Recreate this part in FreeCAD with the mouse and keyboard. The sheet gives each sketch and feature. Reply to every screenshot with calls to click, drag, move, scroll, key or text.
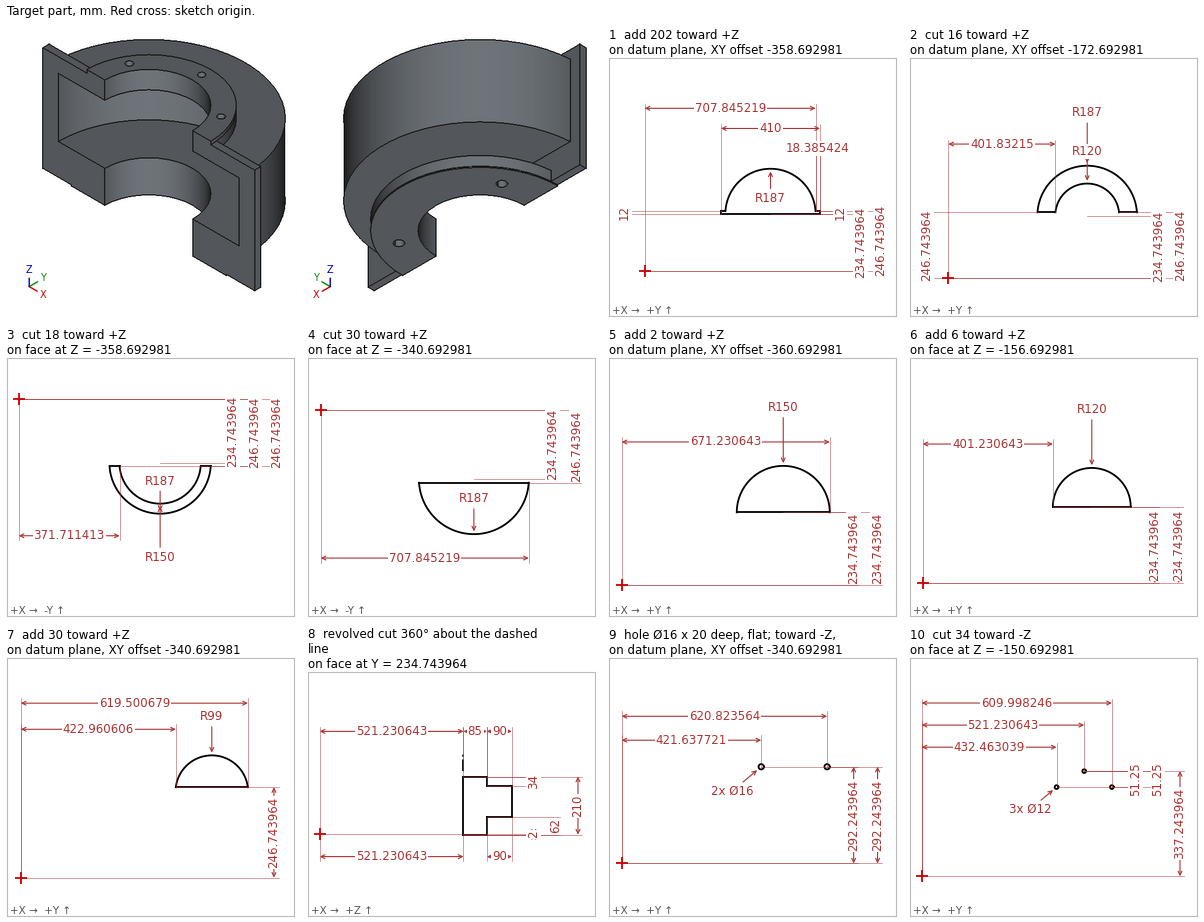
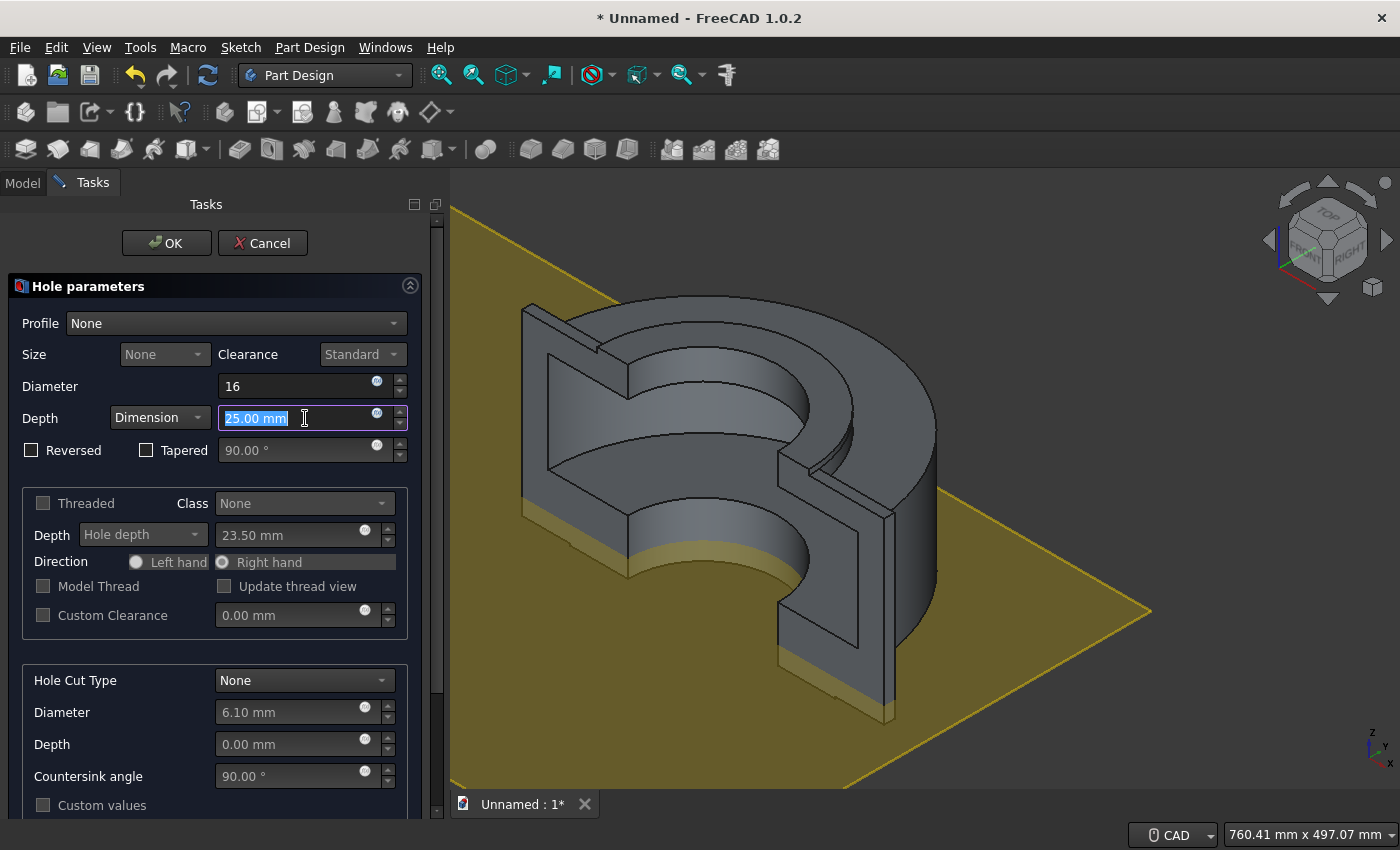
text(20)
key(Tab)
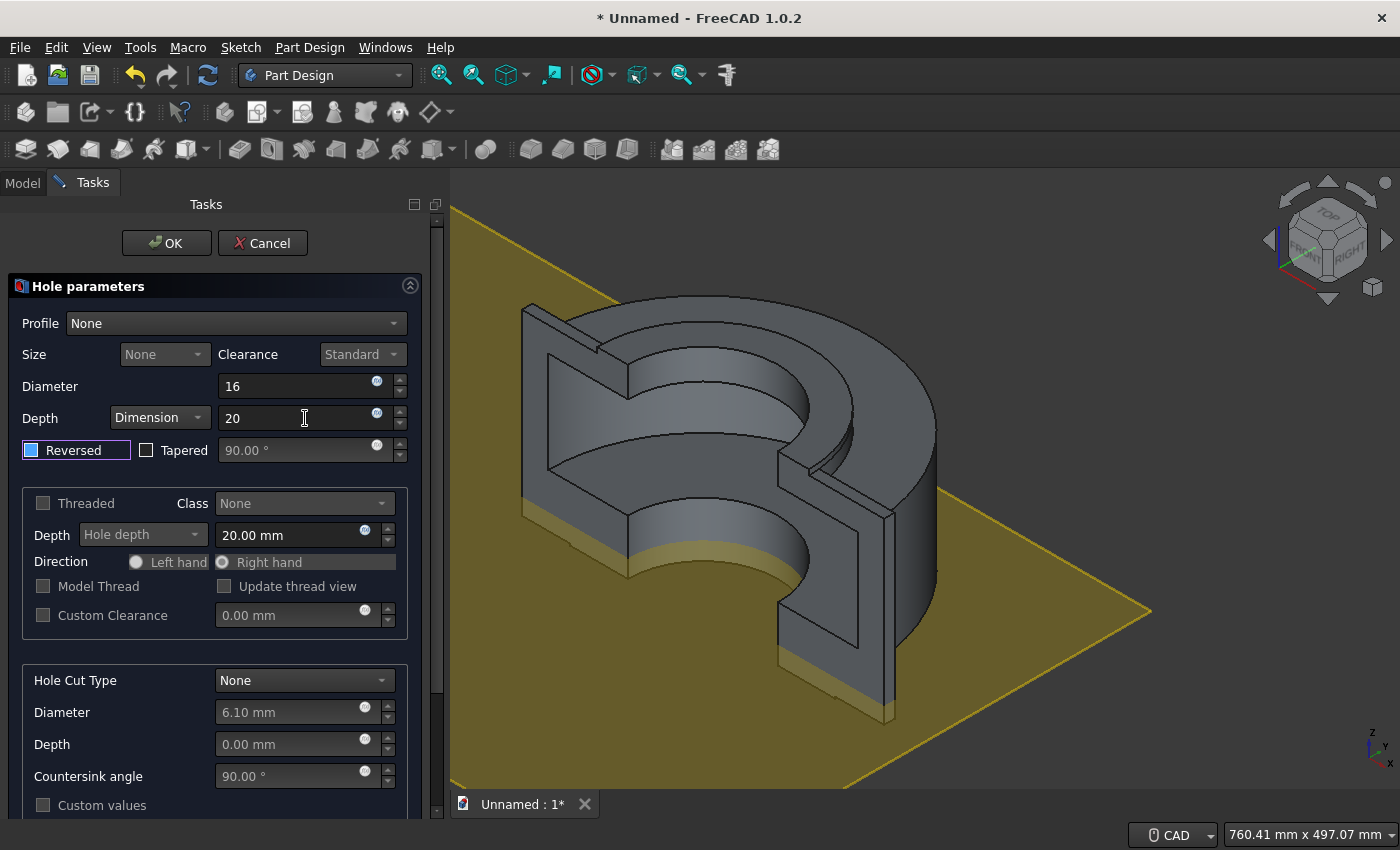
scroll(437, 516, down, 2)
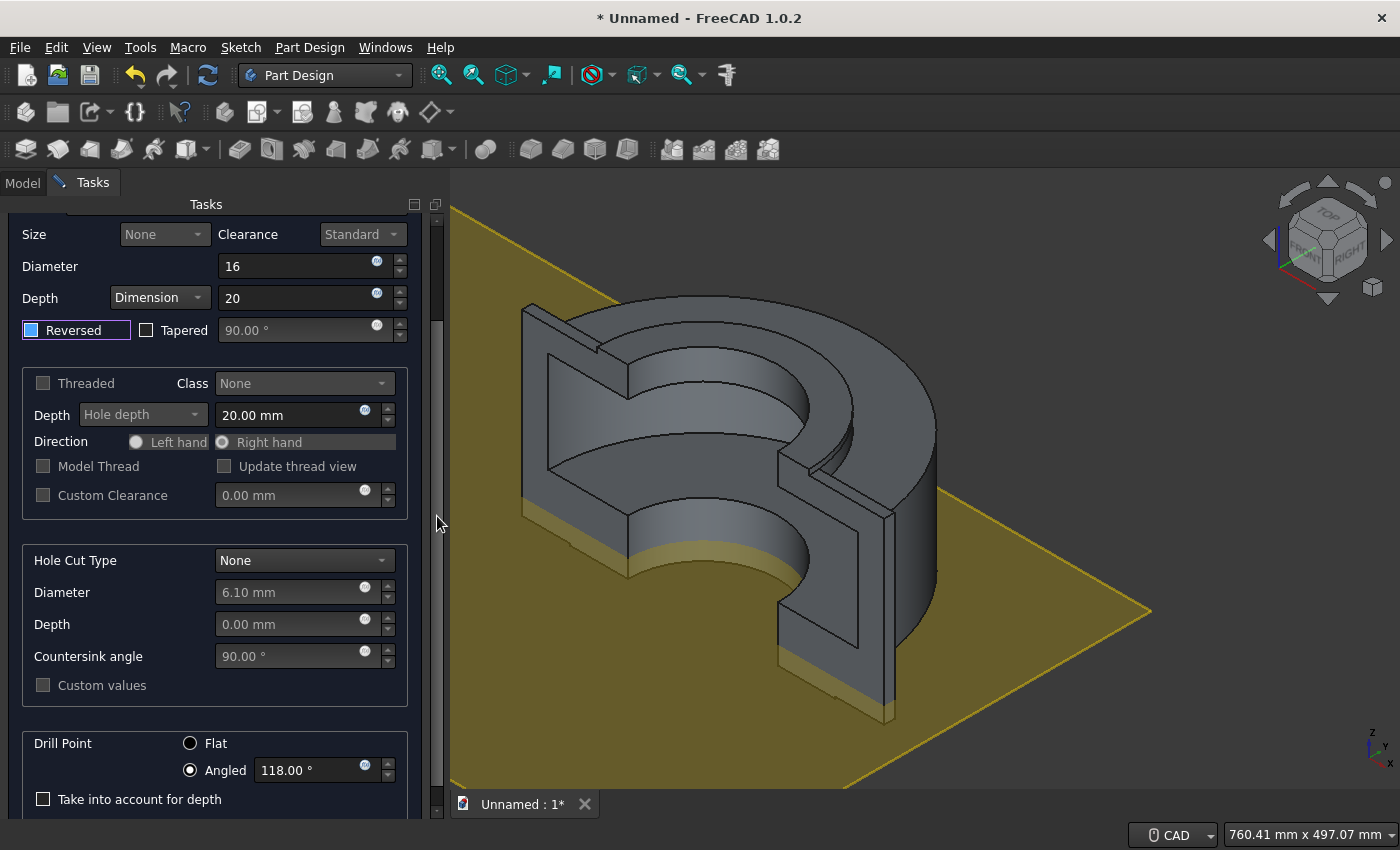
click(191, 743)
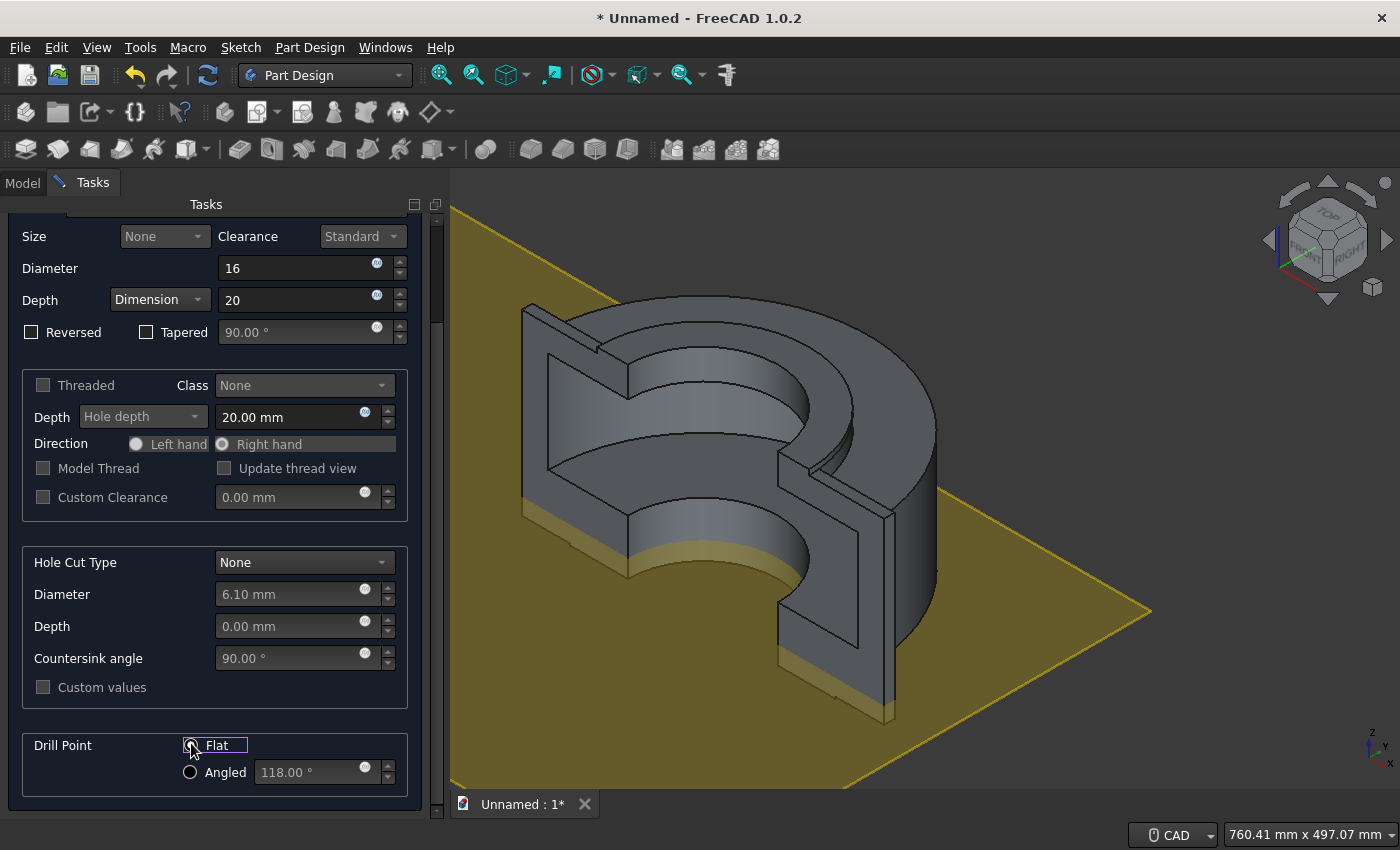
scroll(437, 516, up, 3)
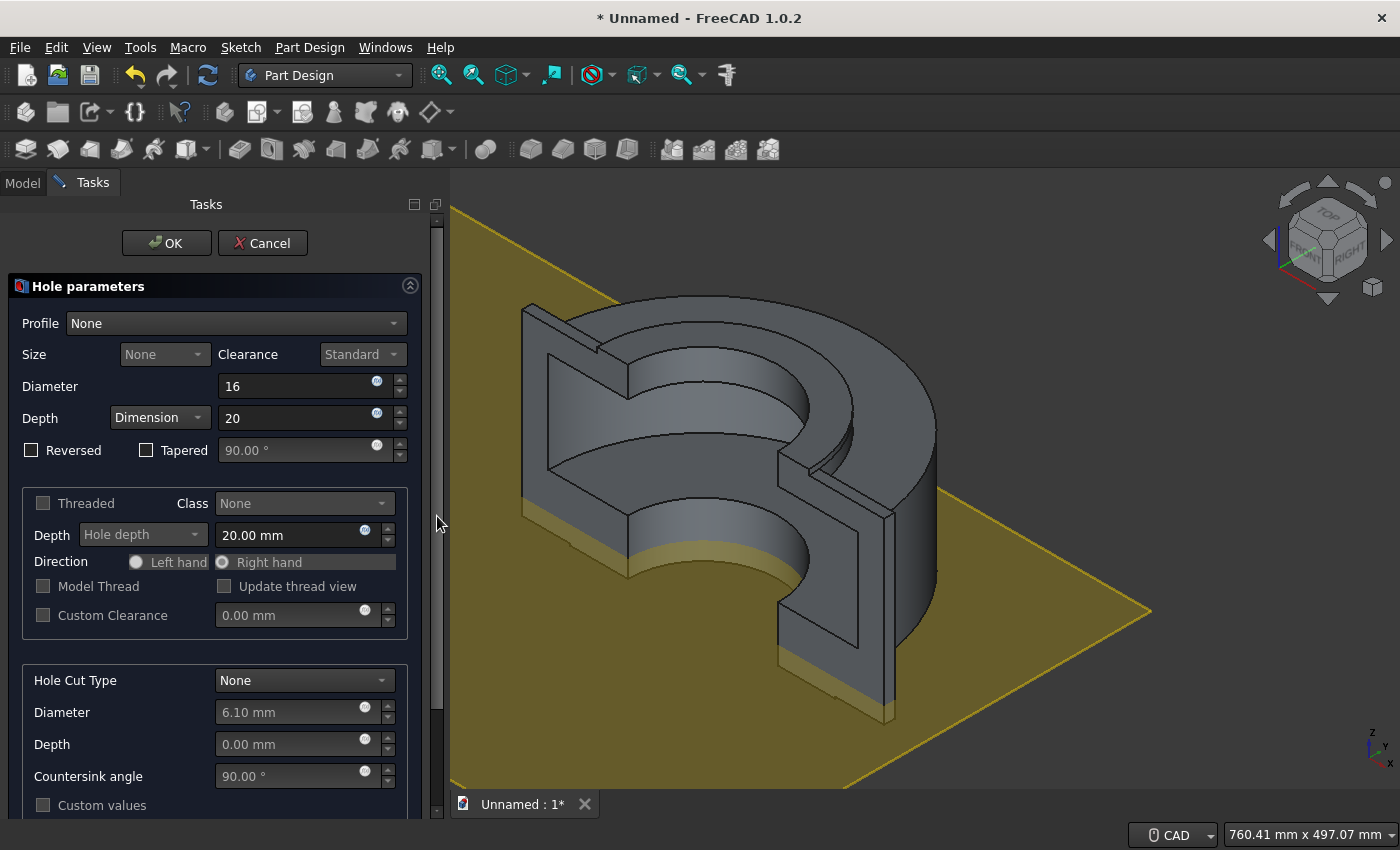
click(167, 243)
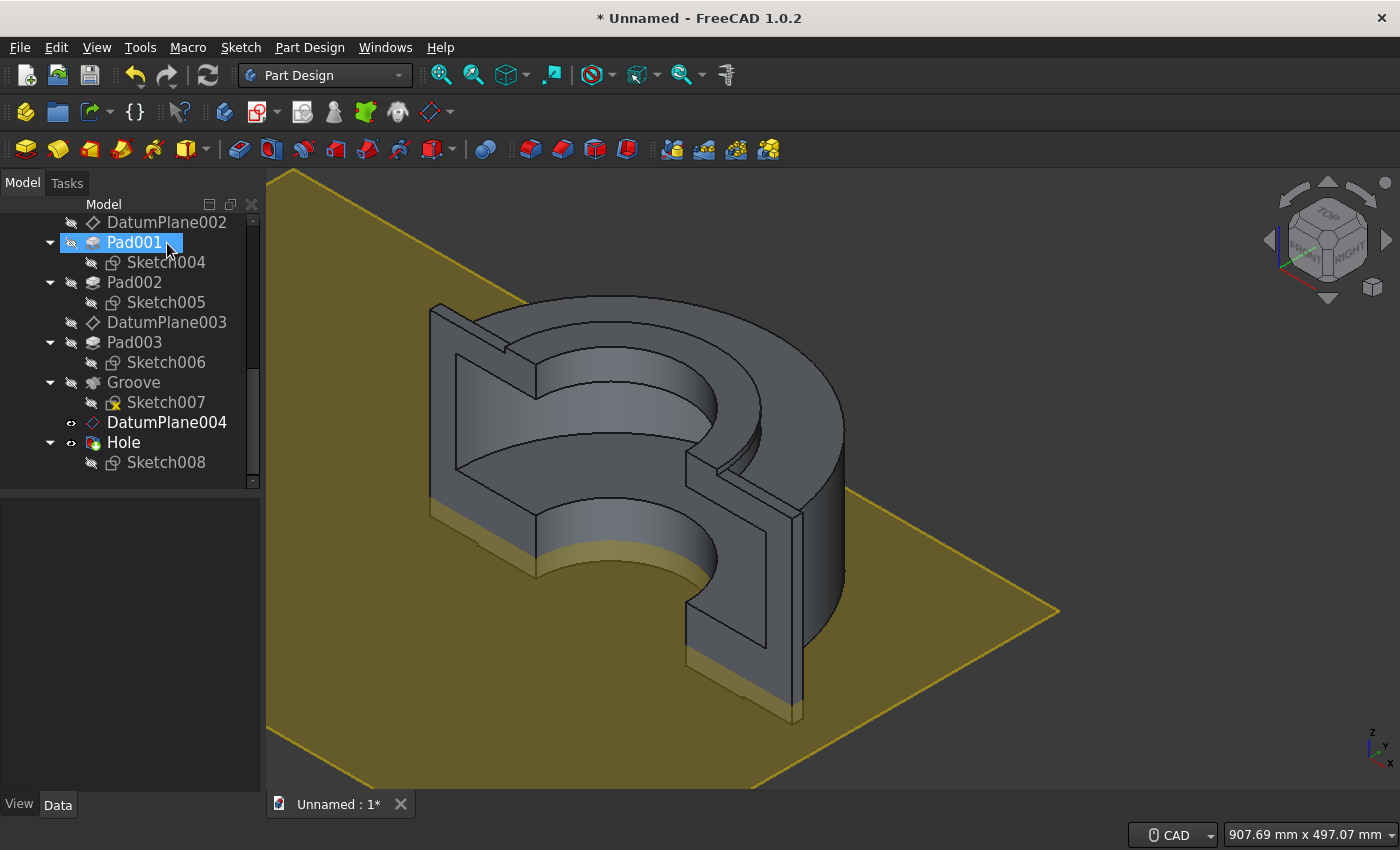
click(116, 423)
key(space)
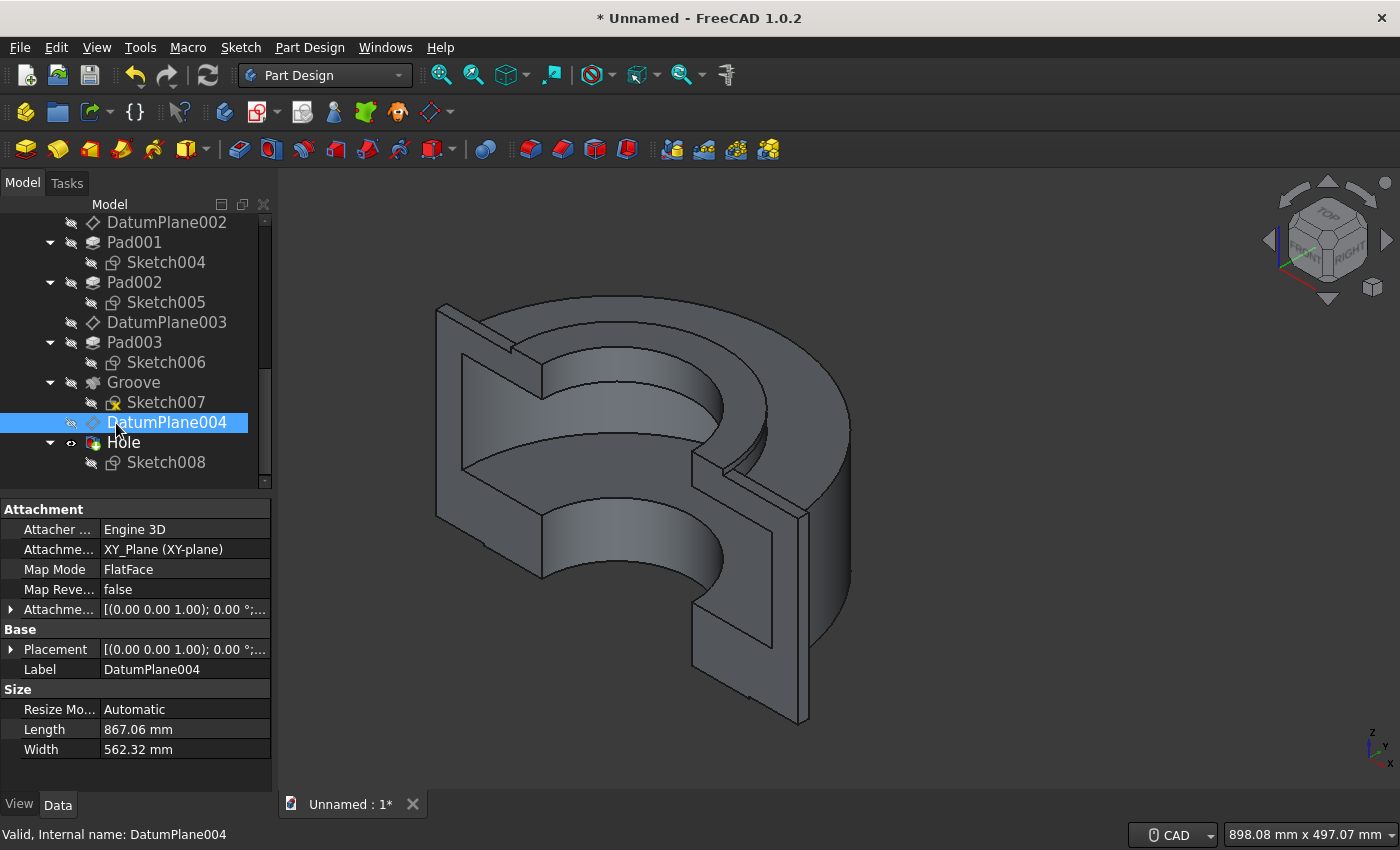
click(746, 403)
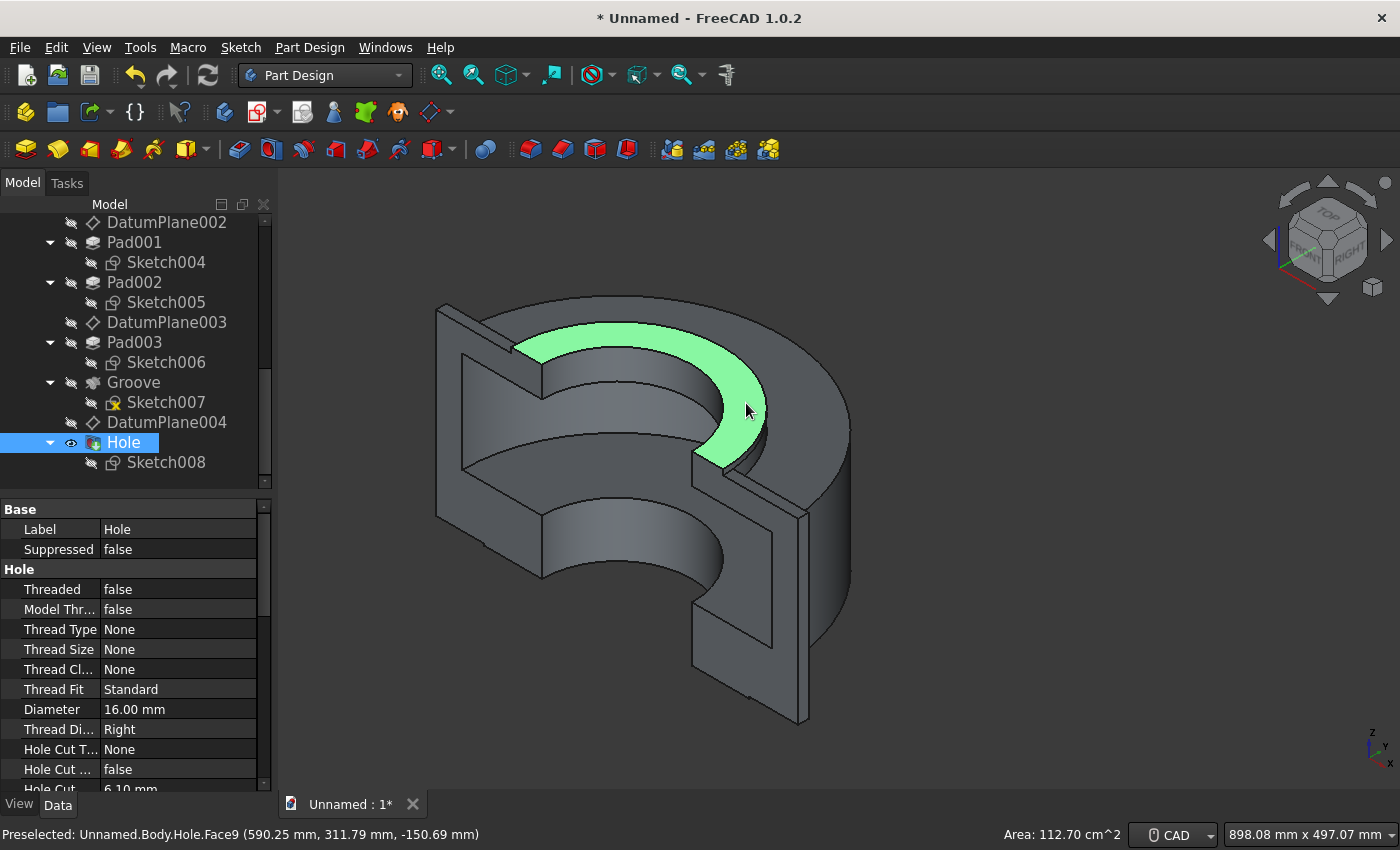
click(258, 112)